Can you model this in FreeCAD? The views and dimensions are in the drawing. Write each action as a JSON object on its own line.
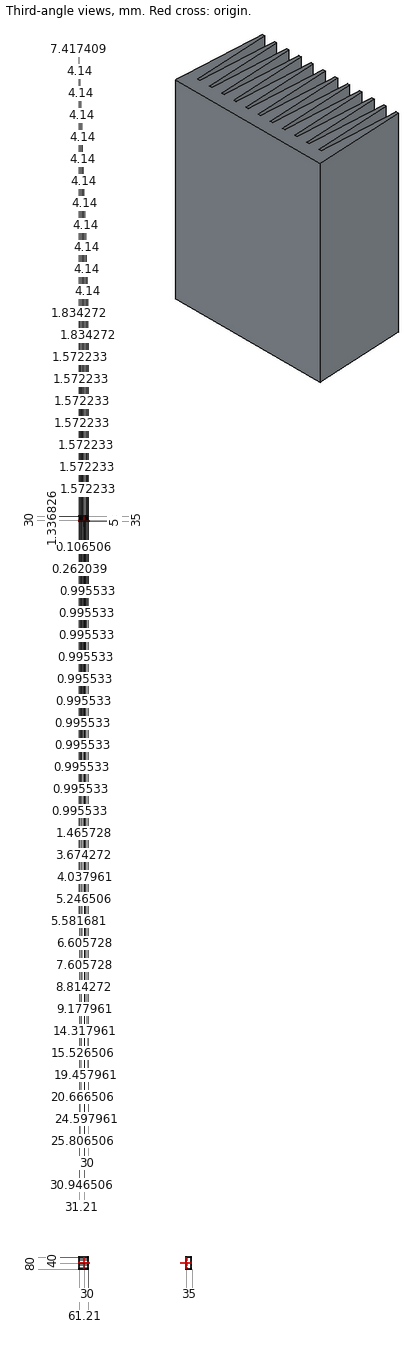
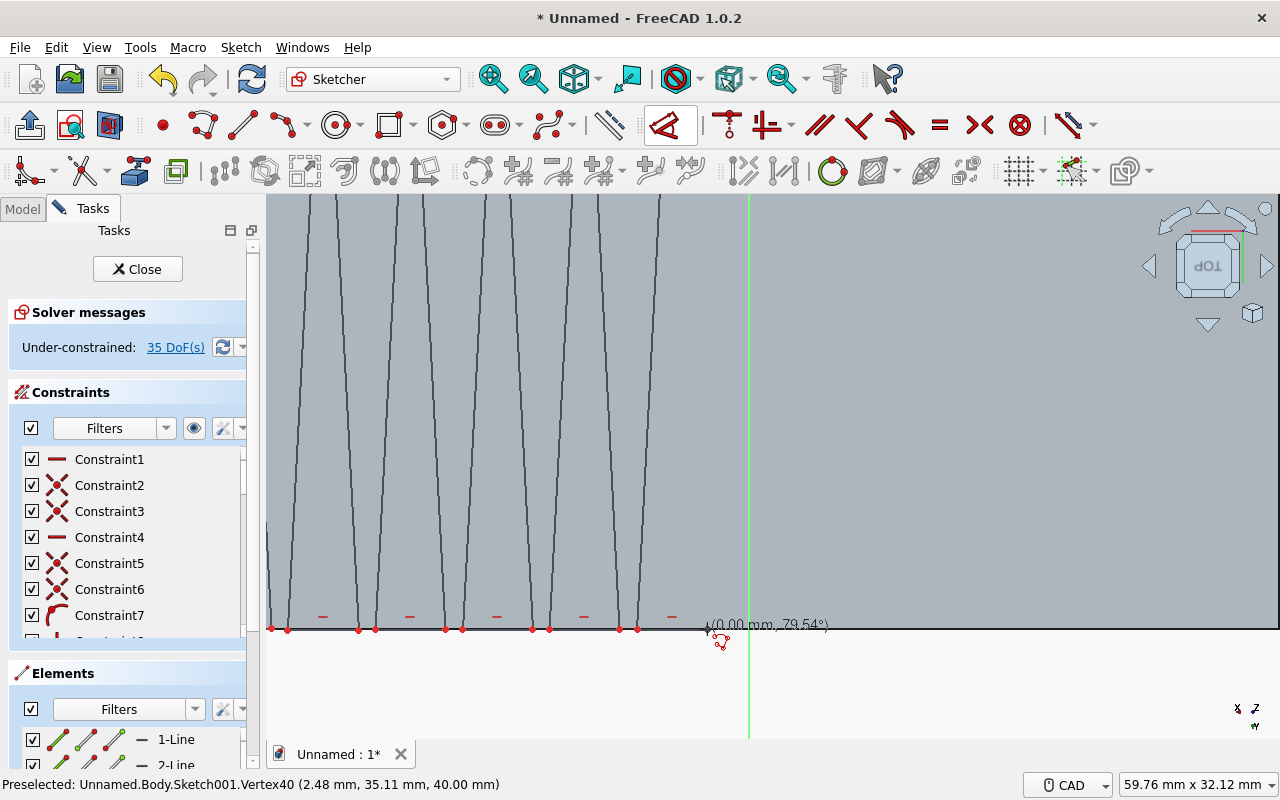
{"action": "scroll", "coordinate": [638, 630], "scroll_direction": "down", "scroll_amount": 3}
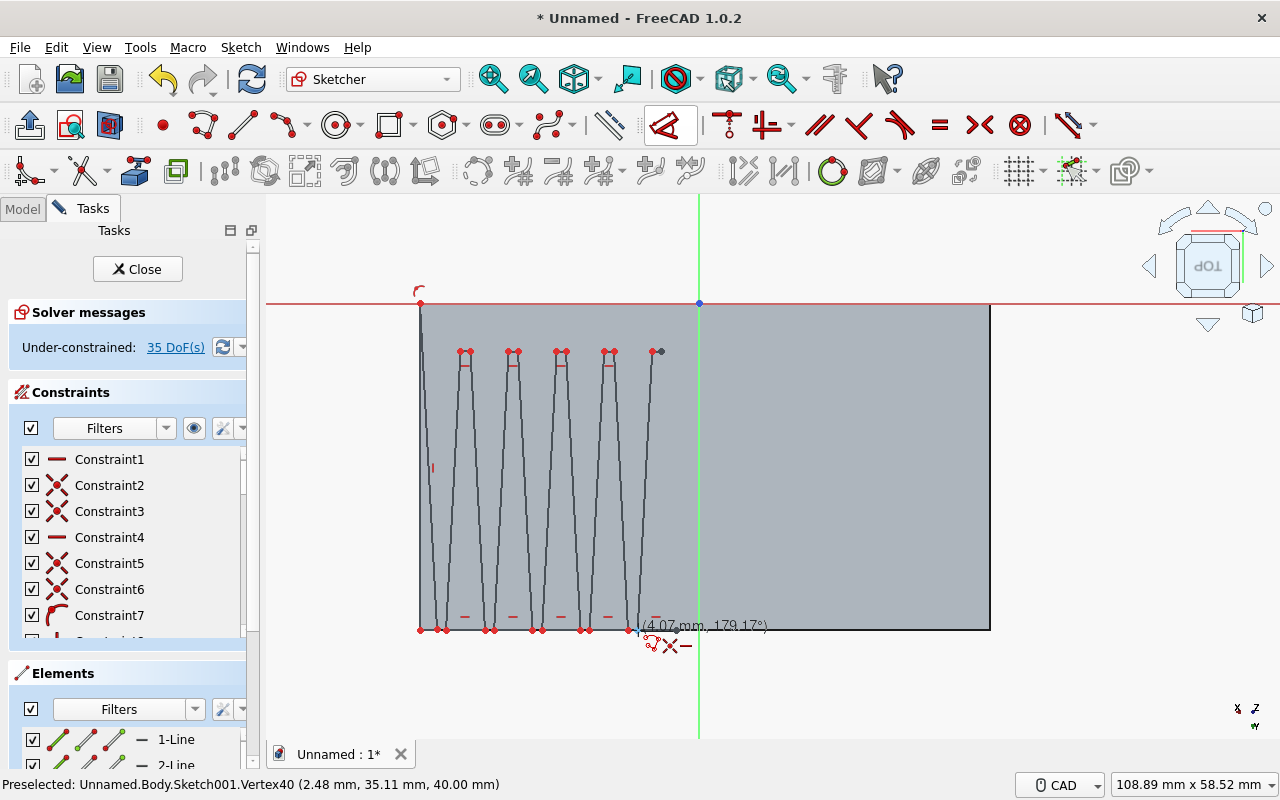
{"action": "scroll", "coordinate": [661, 351], "scroll_direction": "up", "scroll_amount": 7}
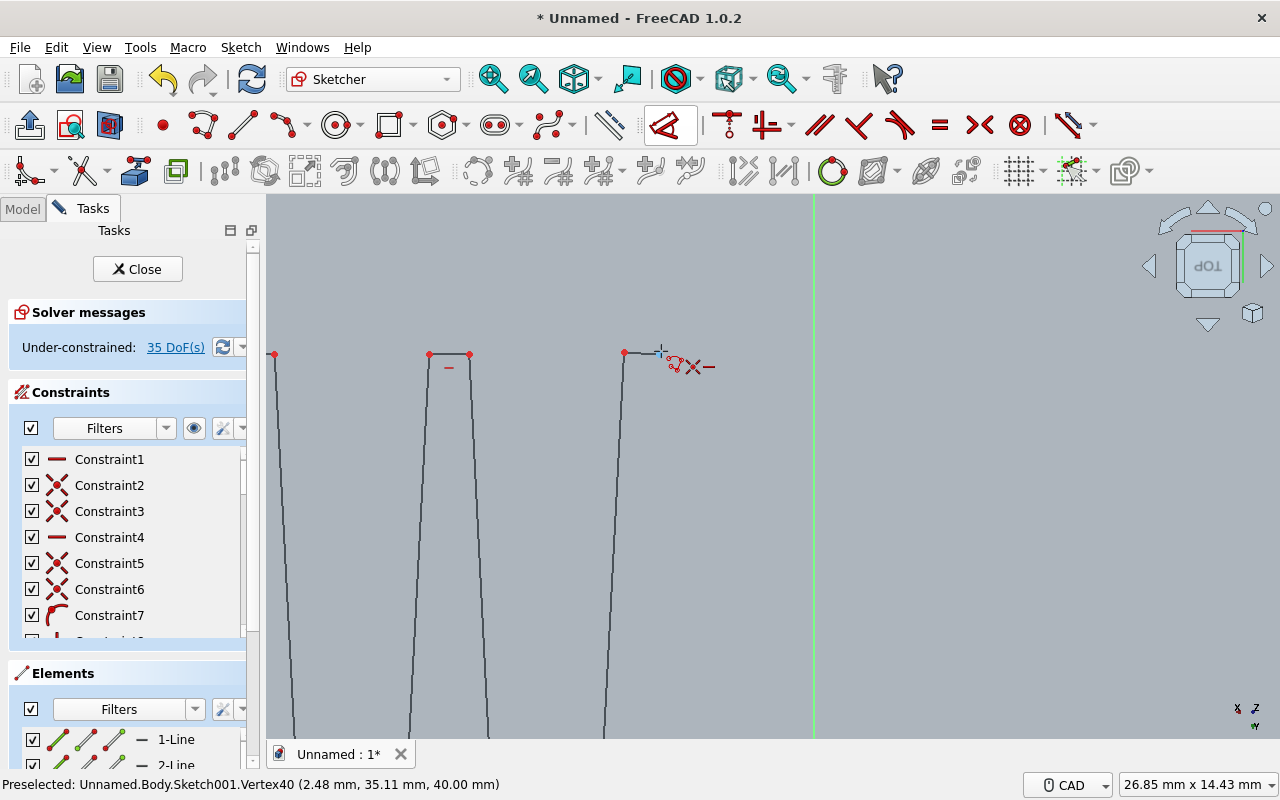
{"action": "left_click", "coordinate": [660, 354]}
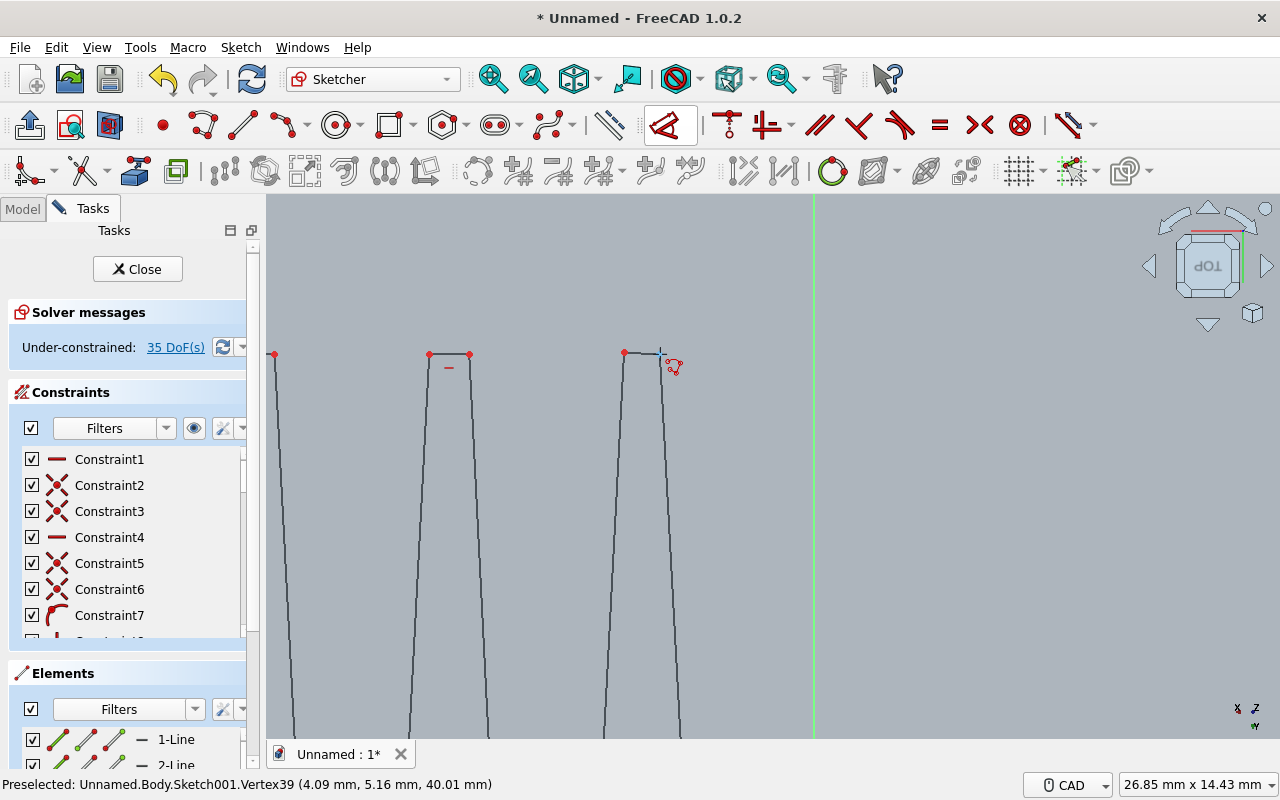
{"action": "scroll", "coordinate": [818, 348], "scroll_direction": "up", "scroll_amount": 7}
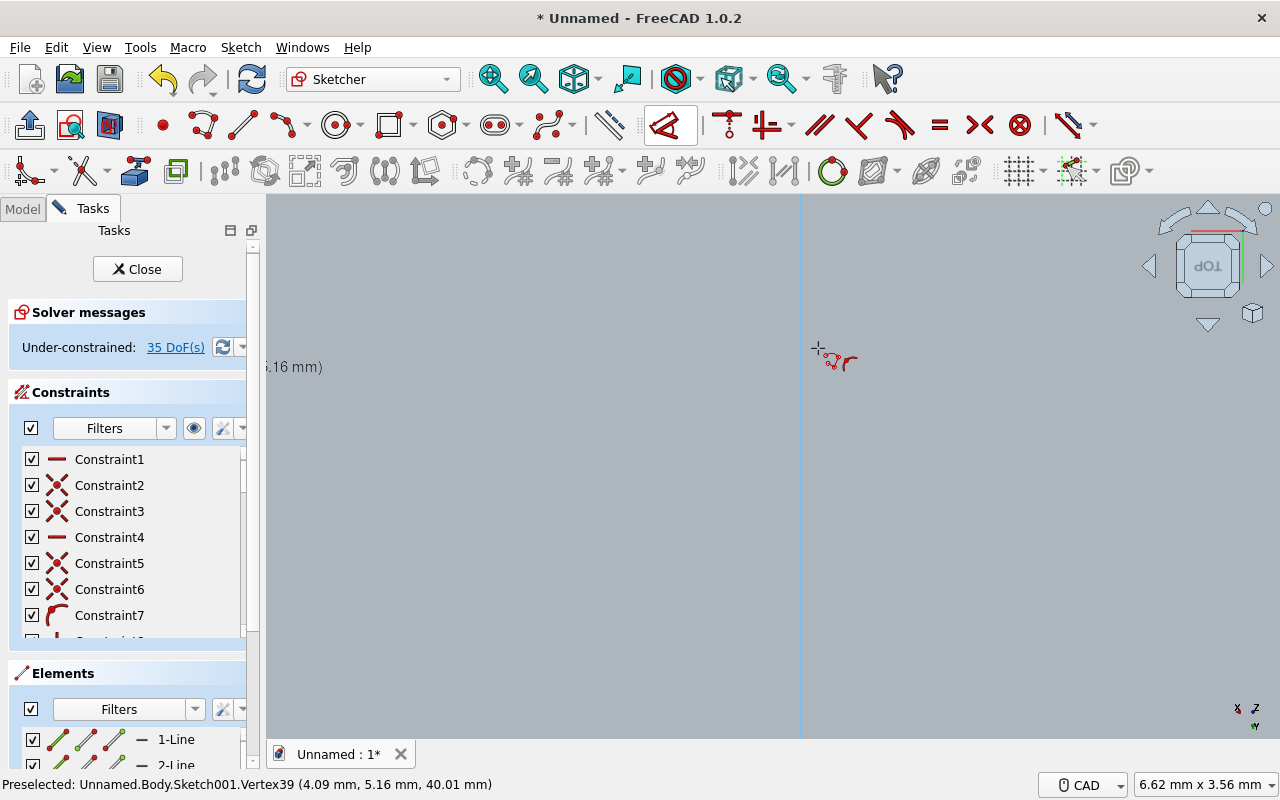
{"action": "left_click", "coordinate": [818, 348]}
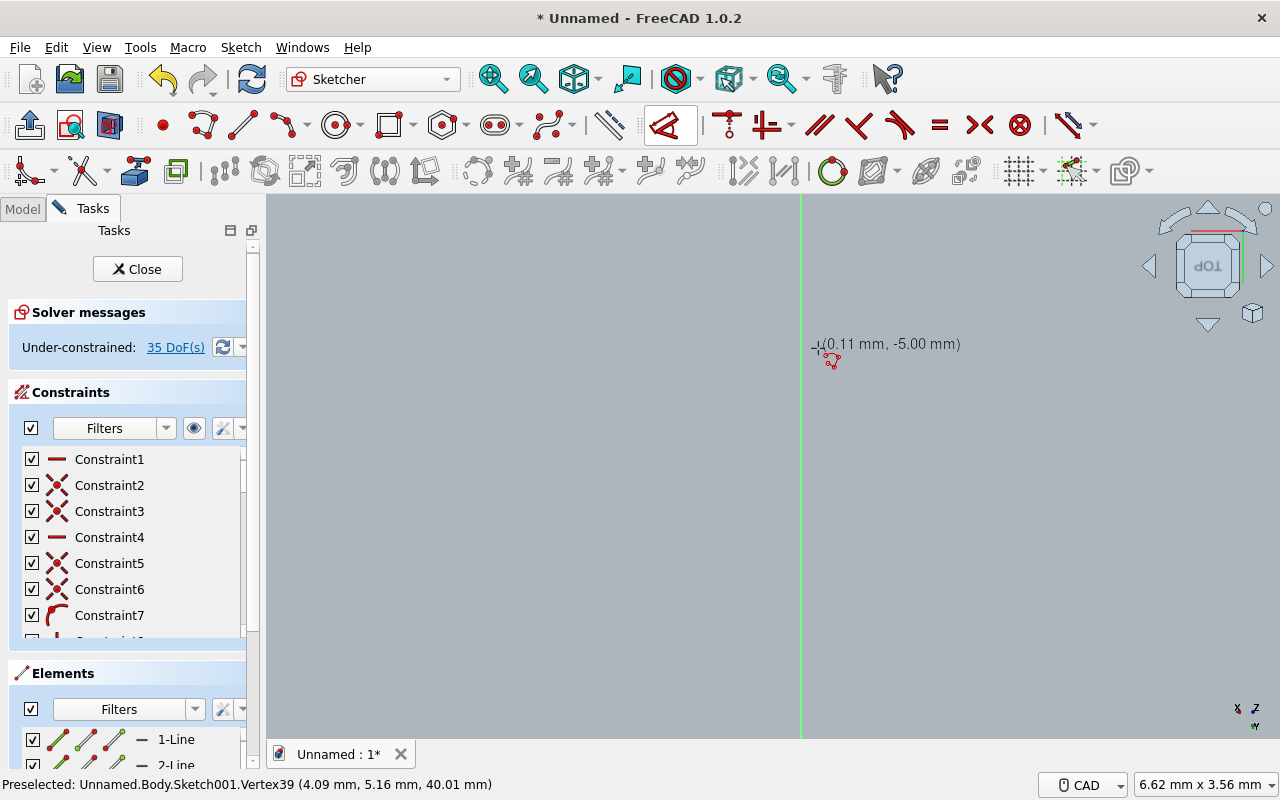
{"action": "scroll", "coordinate": [692, 350], "scroll_direction": "down", "scroll_amount": 14}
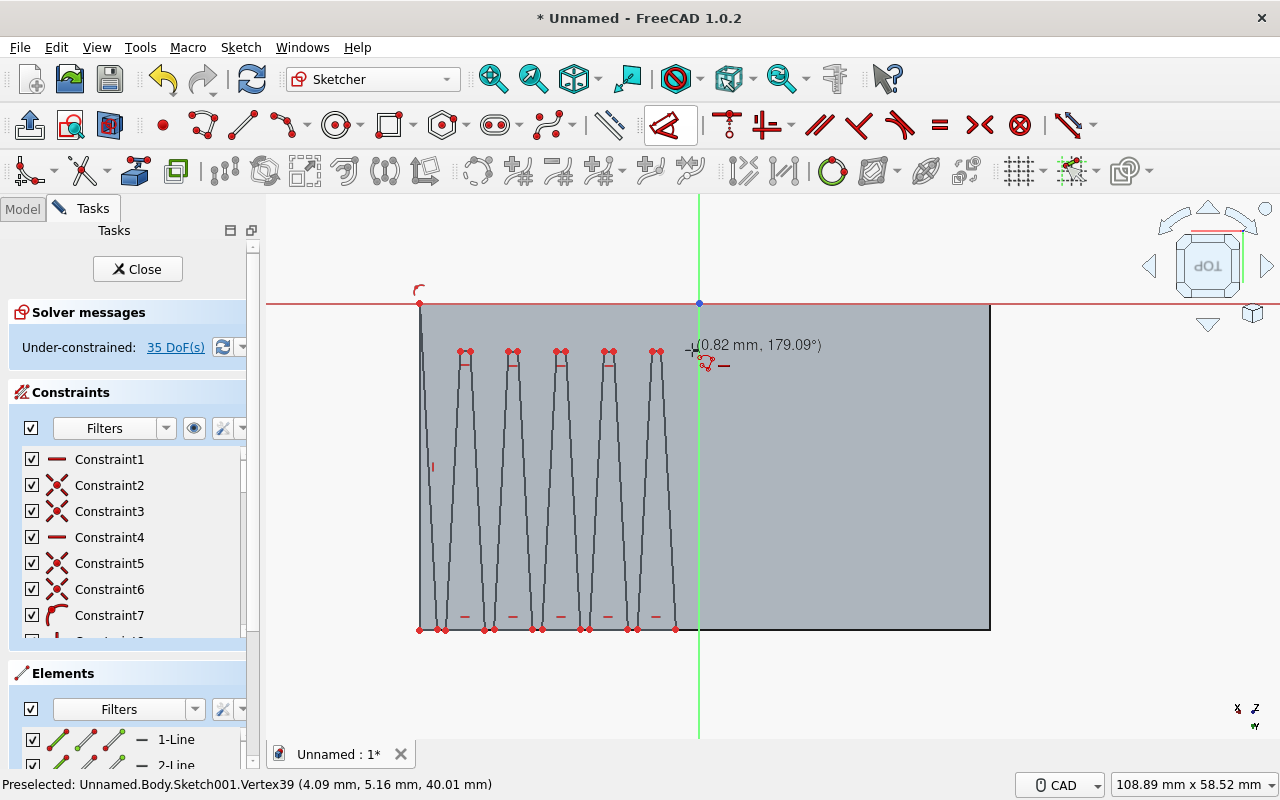
{"action": "scroll", "coordinate": [685, 630], "scroll_direction": "up", "scroll_amount": 3}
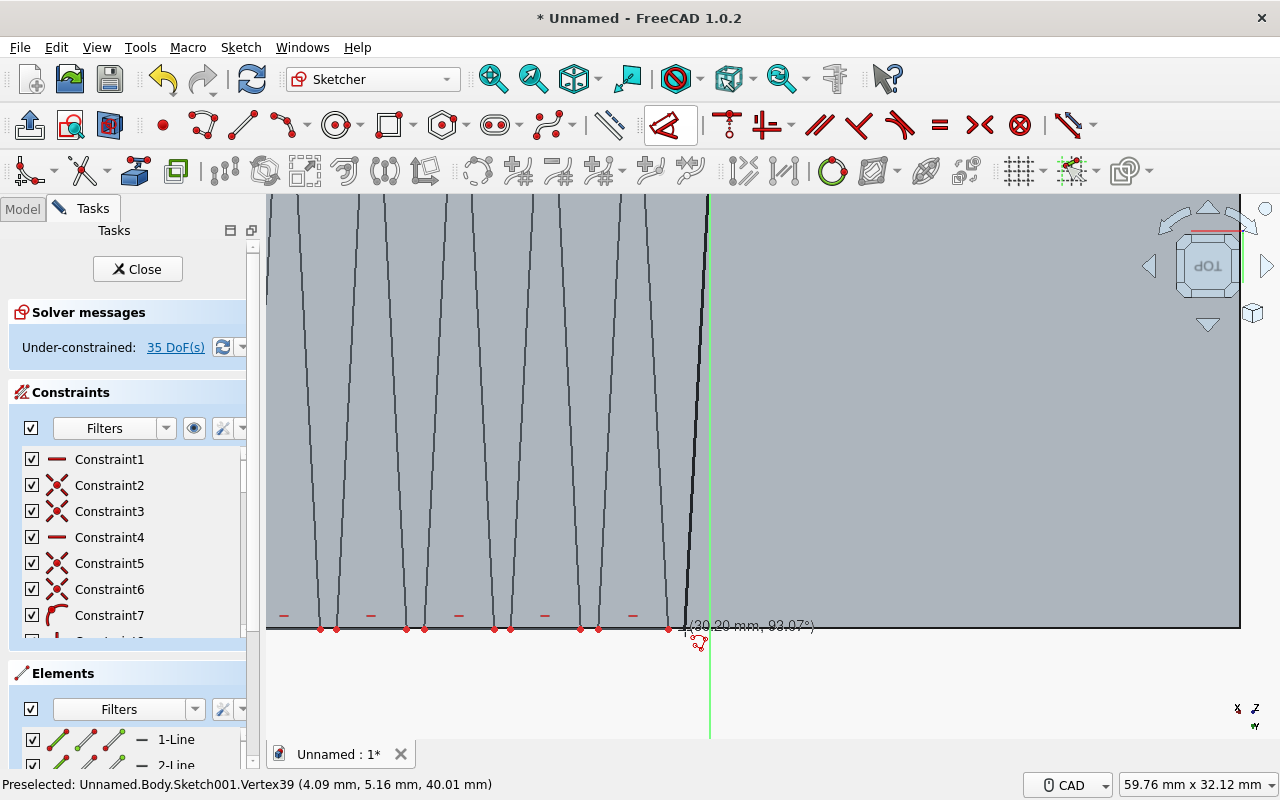
{"action": "left_click", "coordinate": [685, 628]}
{"action": "left_click", "coordinate": [756, 628]}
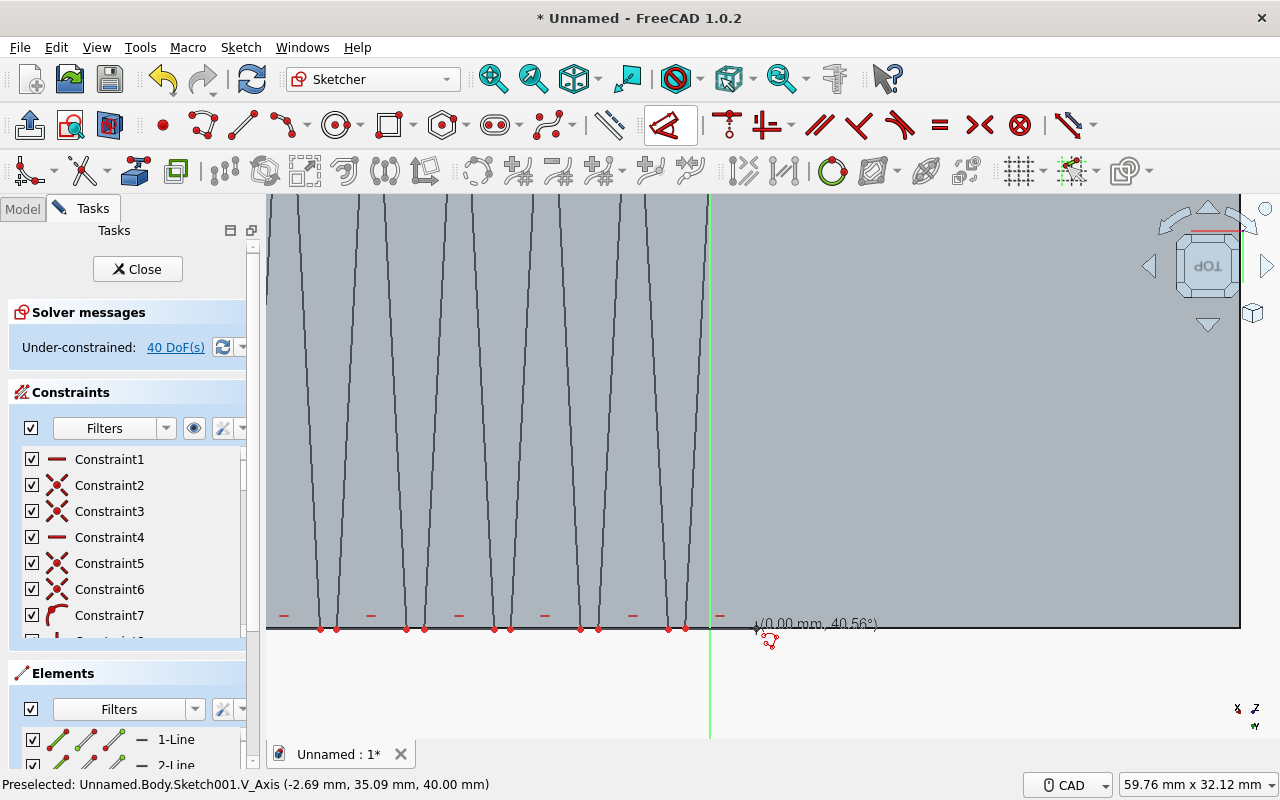
{"action": "scroll", "coordinate": [685, 631], "scroll_direction": "down", "scroll_amount": 3}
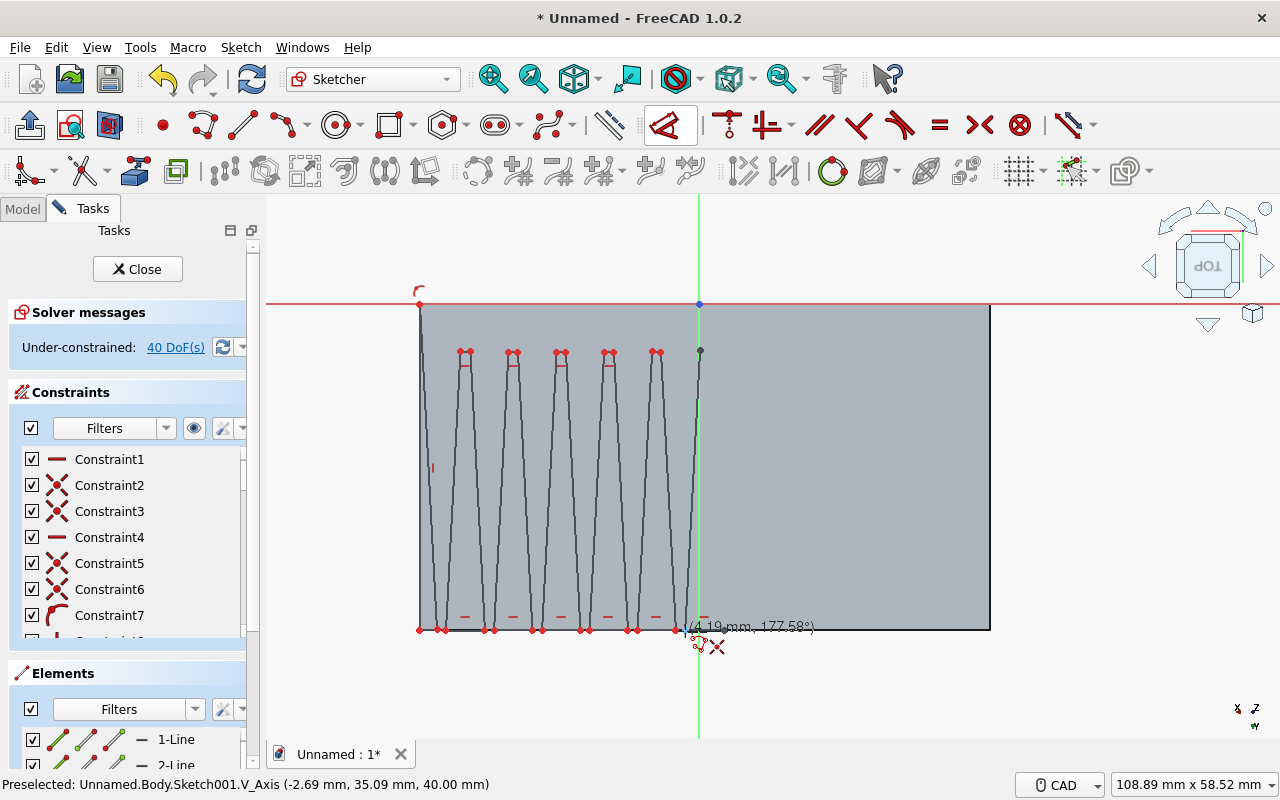
{"action": "scroll", "coordinate": [709, 351], "scroll_direction": "up", "scroll_amount": 3}